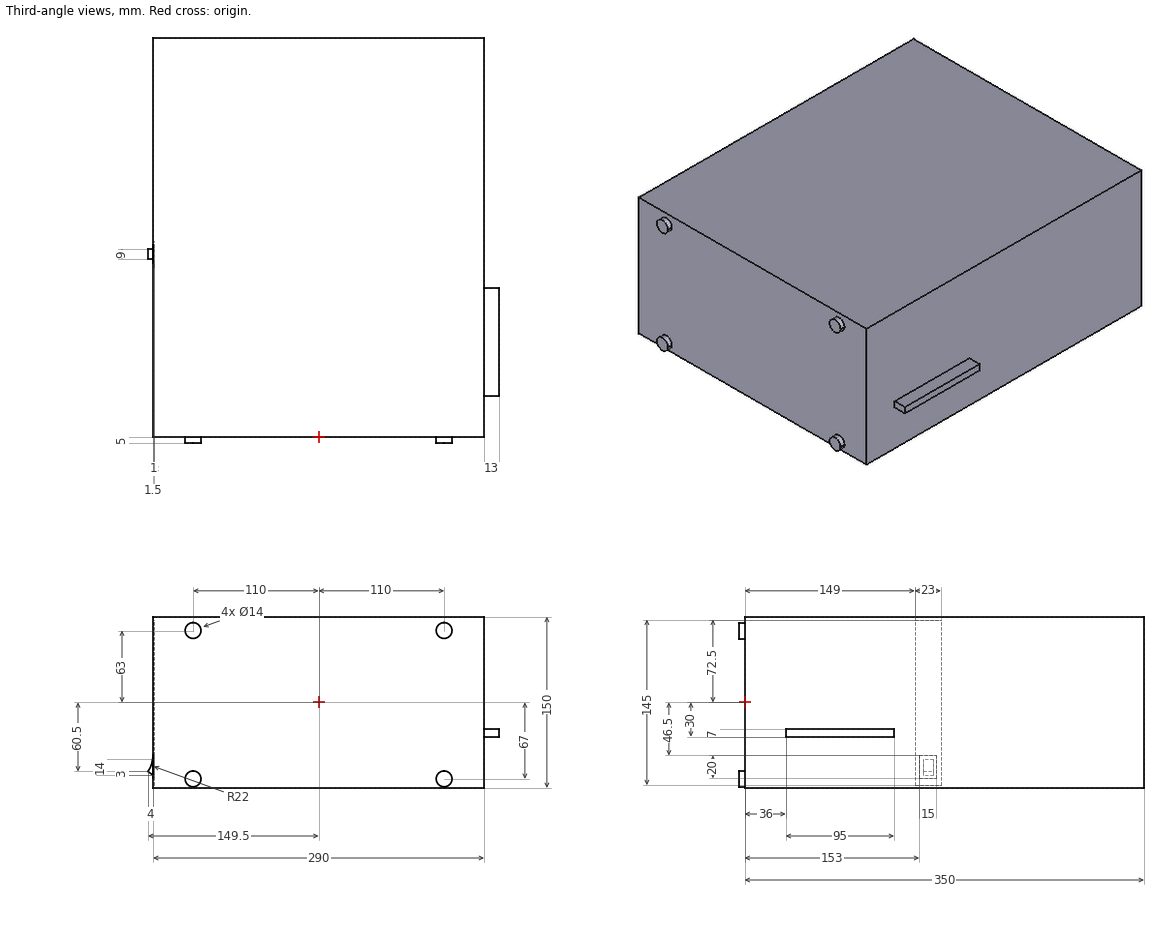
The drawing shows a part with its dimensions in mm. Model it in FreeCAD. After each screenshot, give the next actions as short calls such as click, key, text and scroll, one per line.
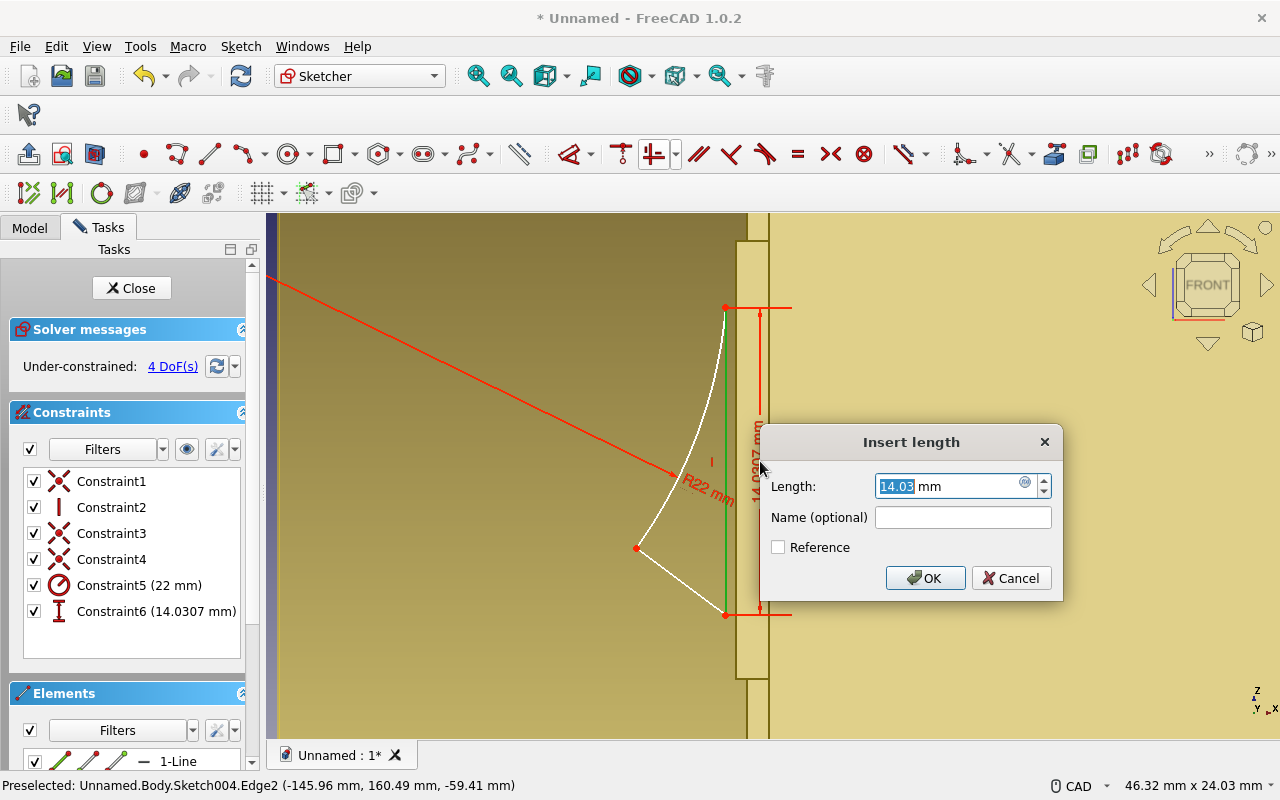
text(14)
key(Return)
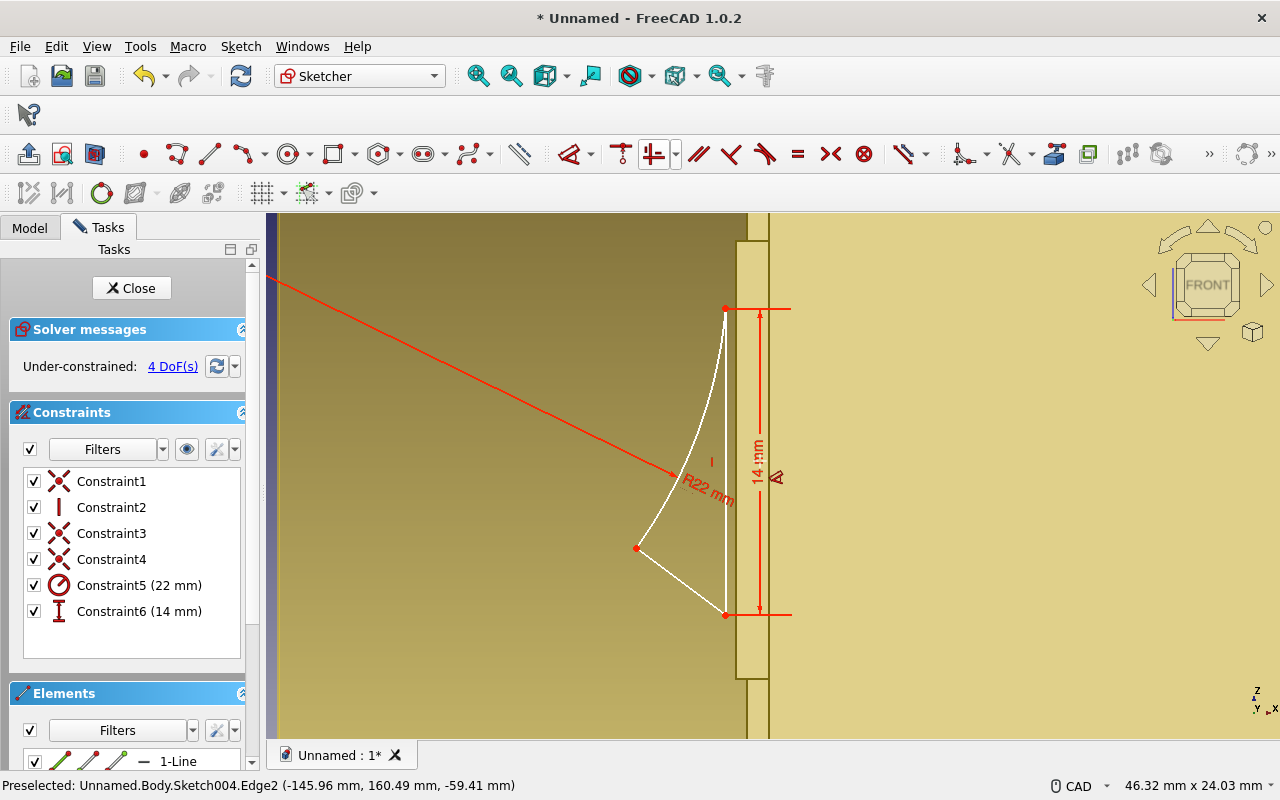
click(663, 568)
click(681, 649)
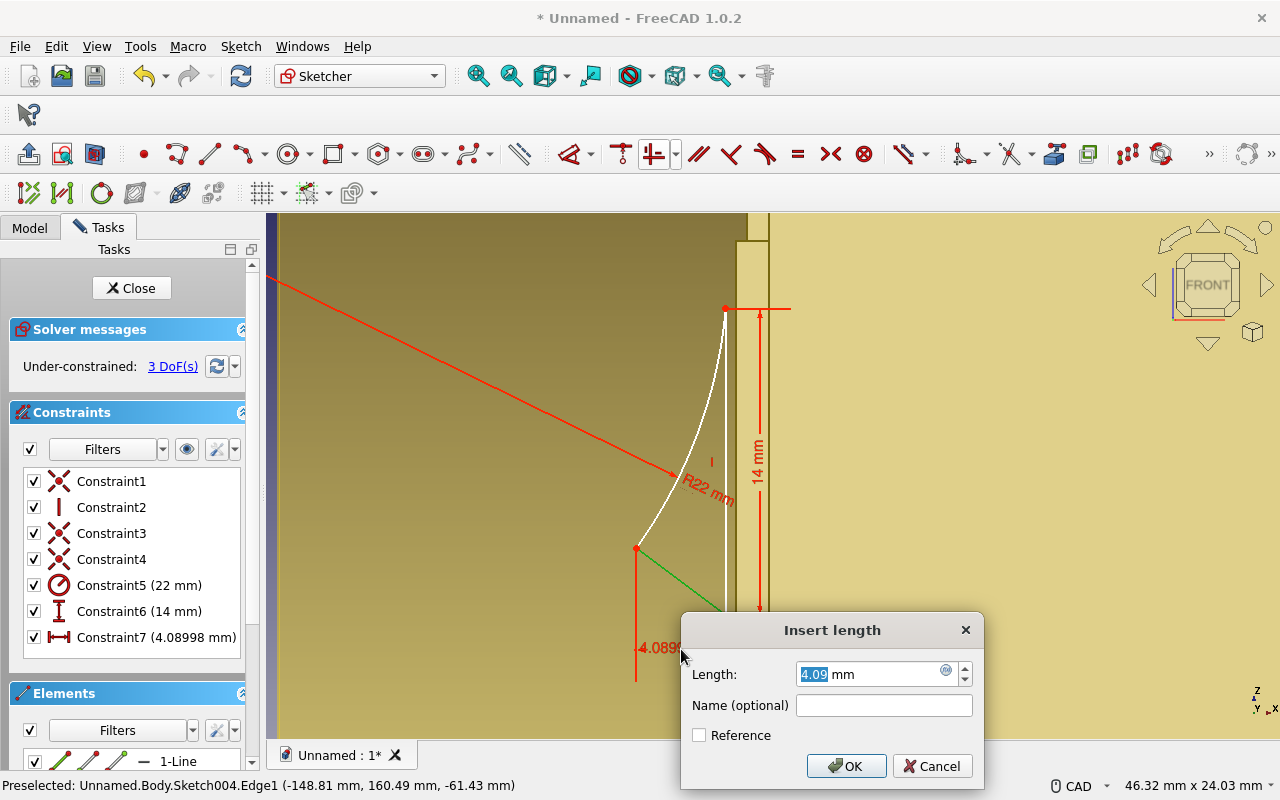
text(4)
key(Return)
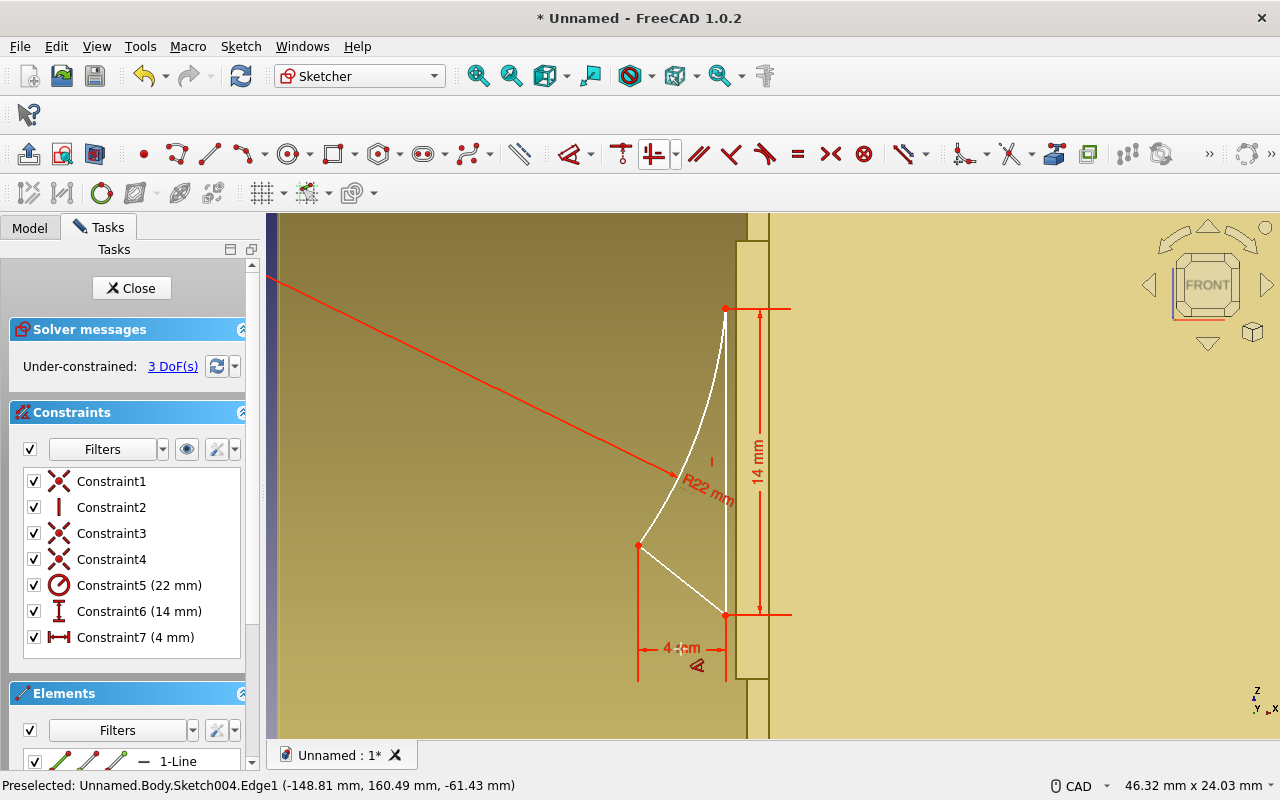
click(665, 566)
click(604, 580)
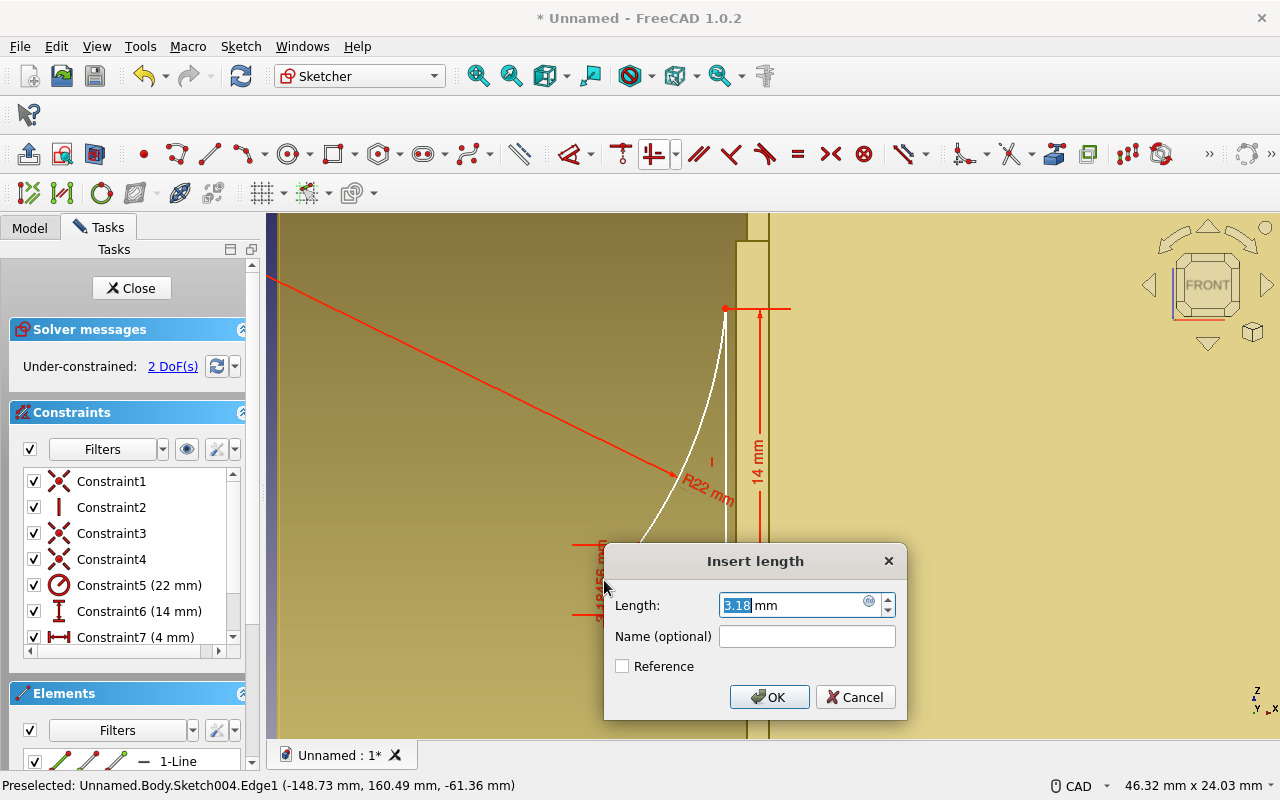
text(3)
key(Return)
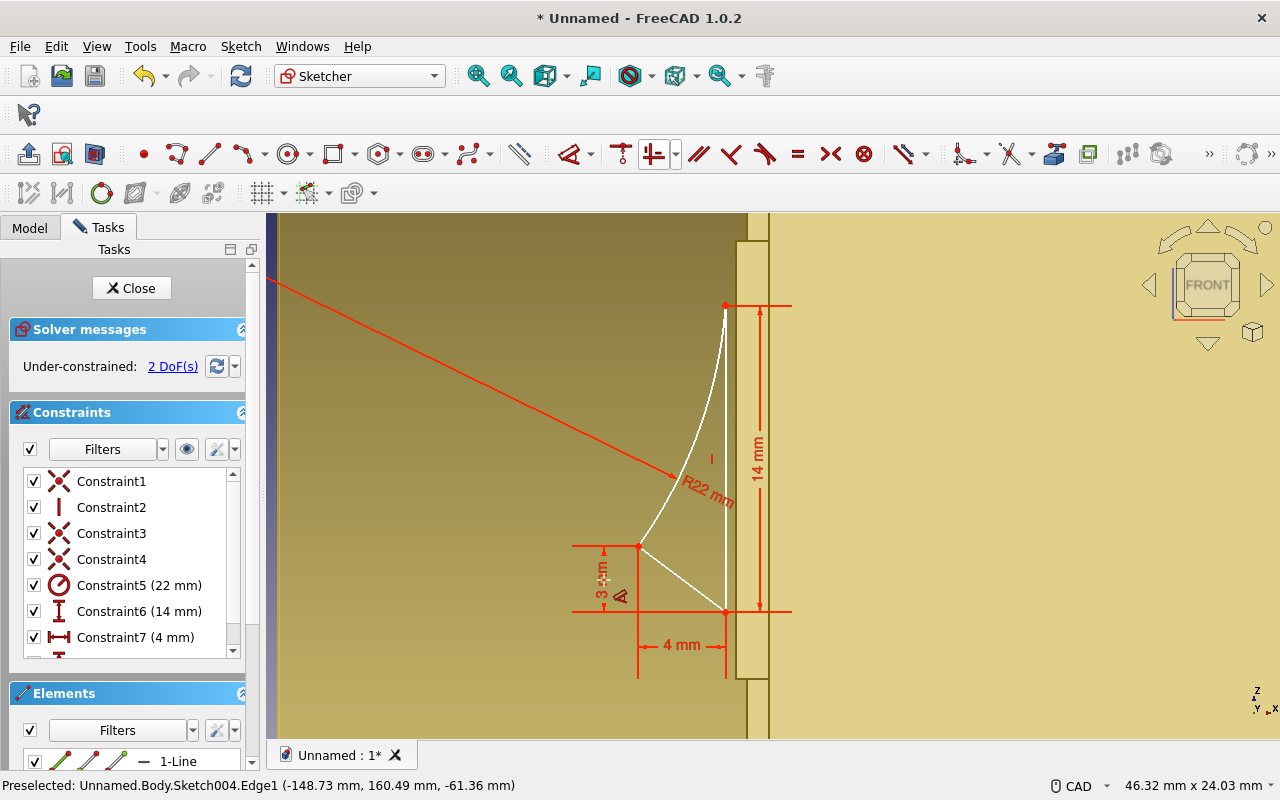
click(638, 546)
click(604, 394)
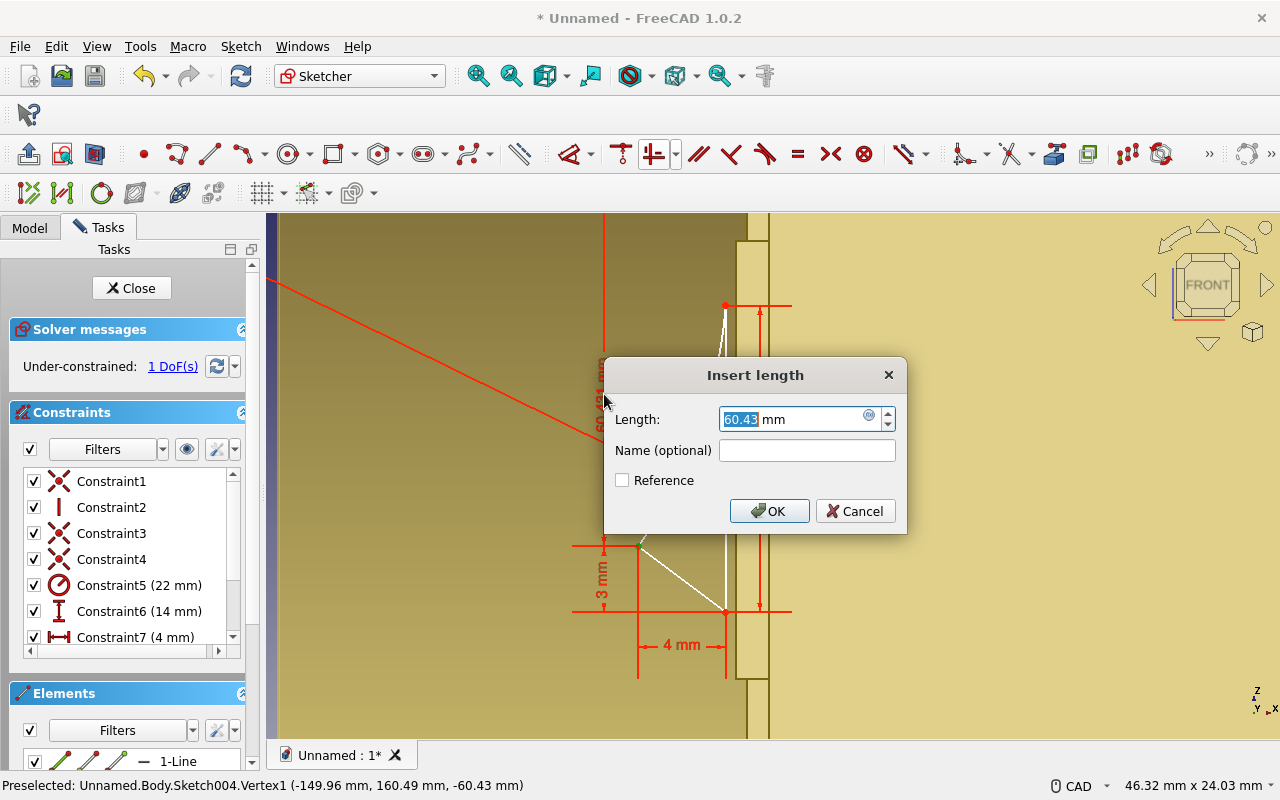
text(60.5)
key(Return)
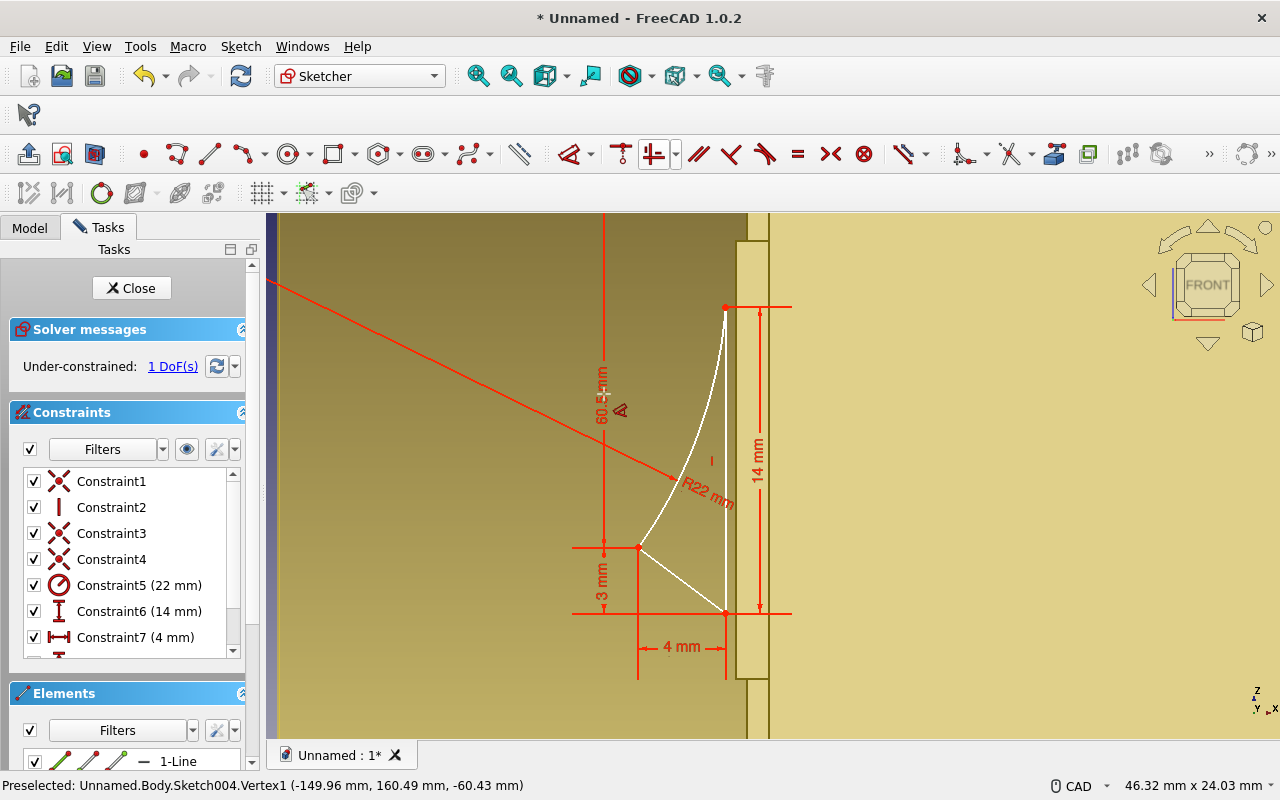
click(638, 548)
click(877, 582)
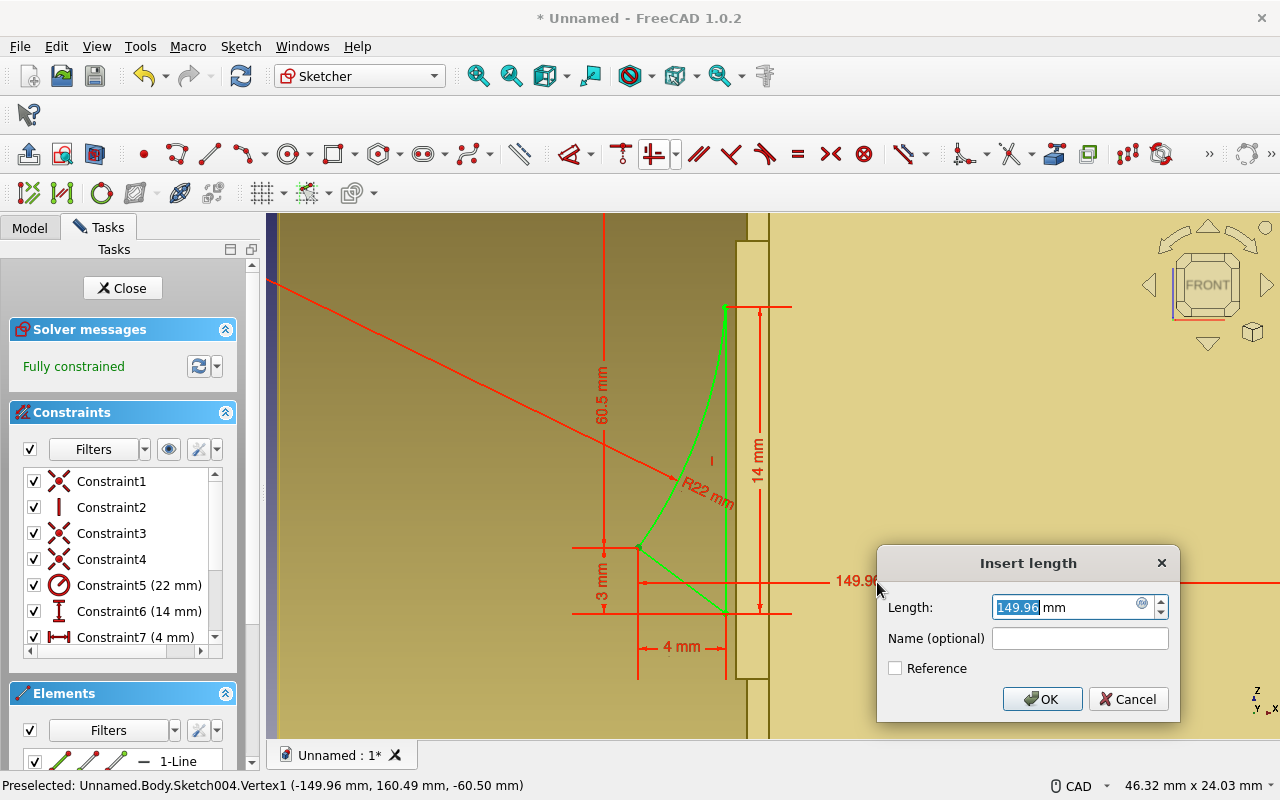
text(149.5)
key(Return)
key(Escape)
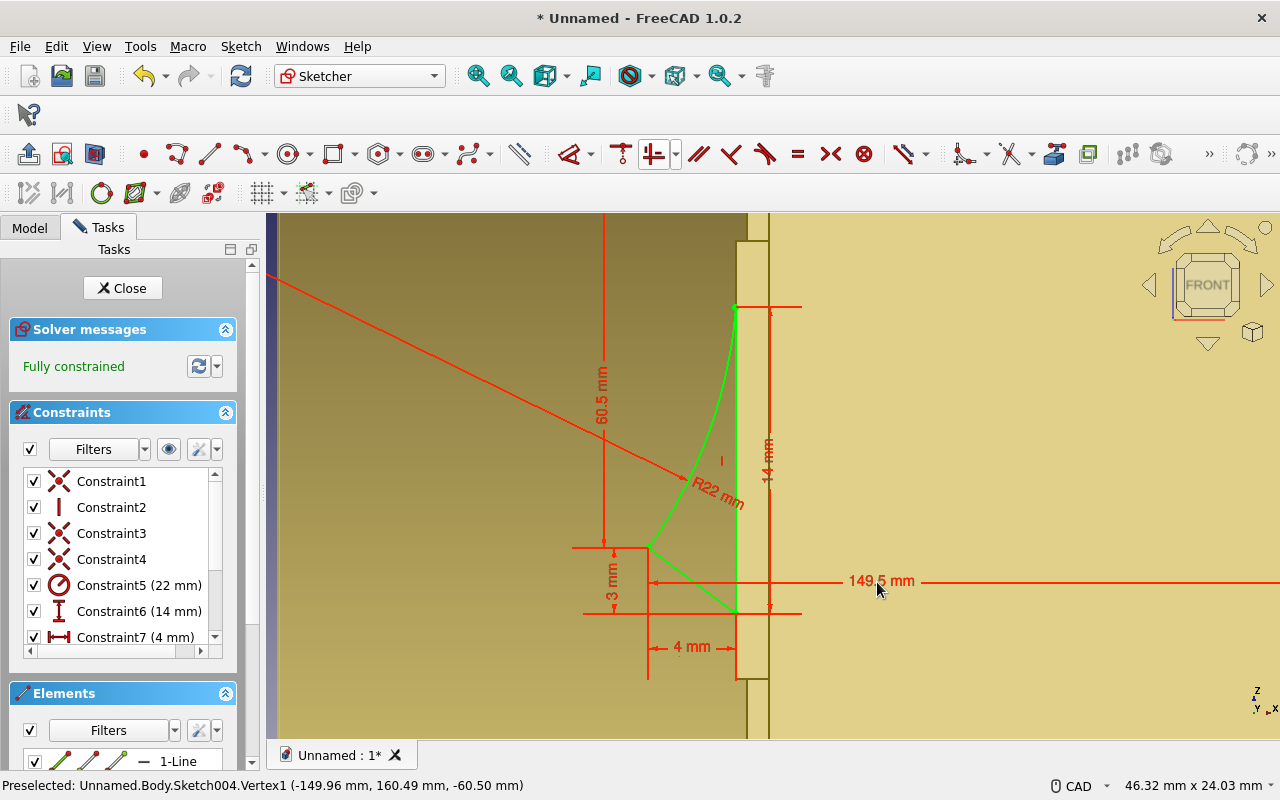
click(123, 288)